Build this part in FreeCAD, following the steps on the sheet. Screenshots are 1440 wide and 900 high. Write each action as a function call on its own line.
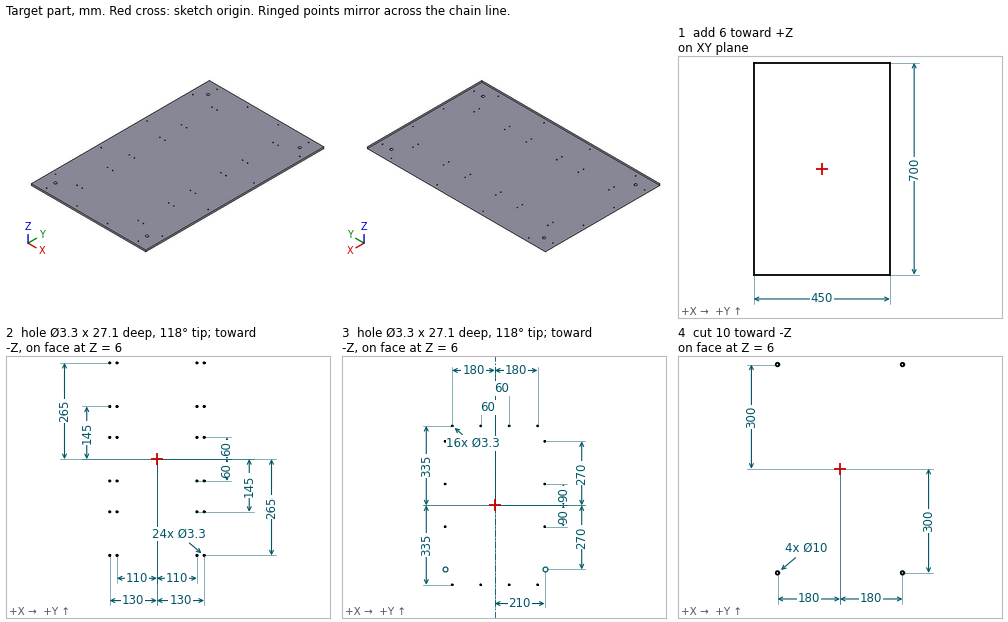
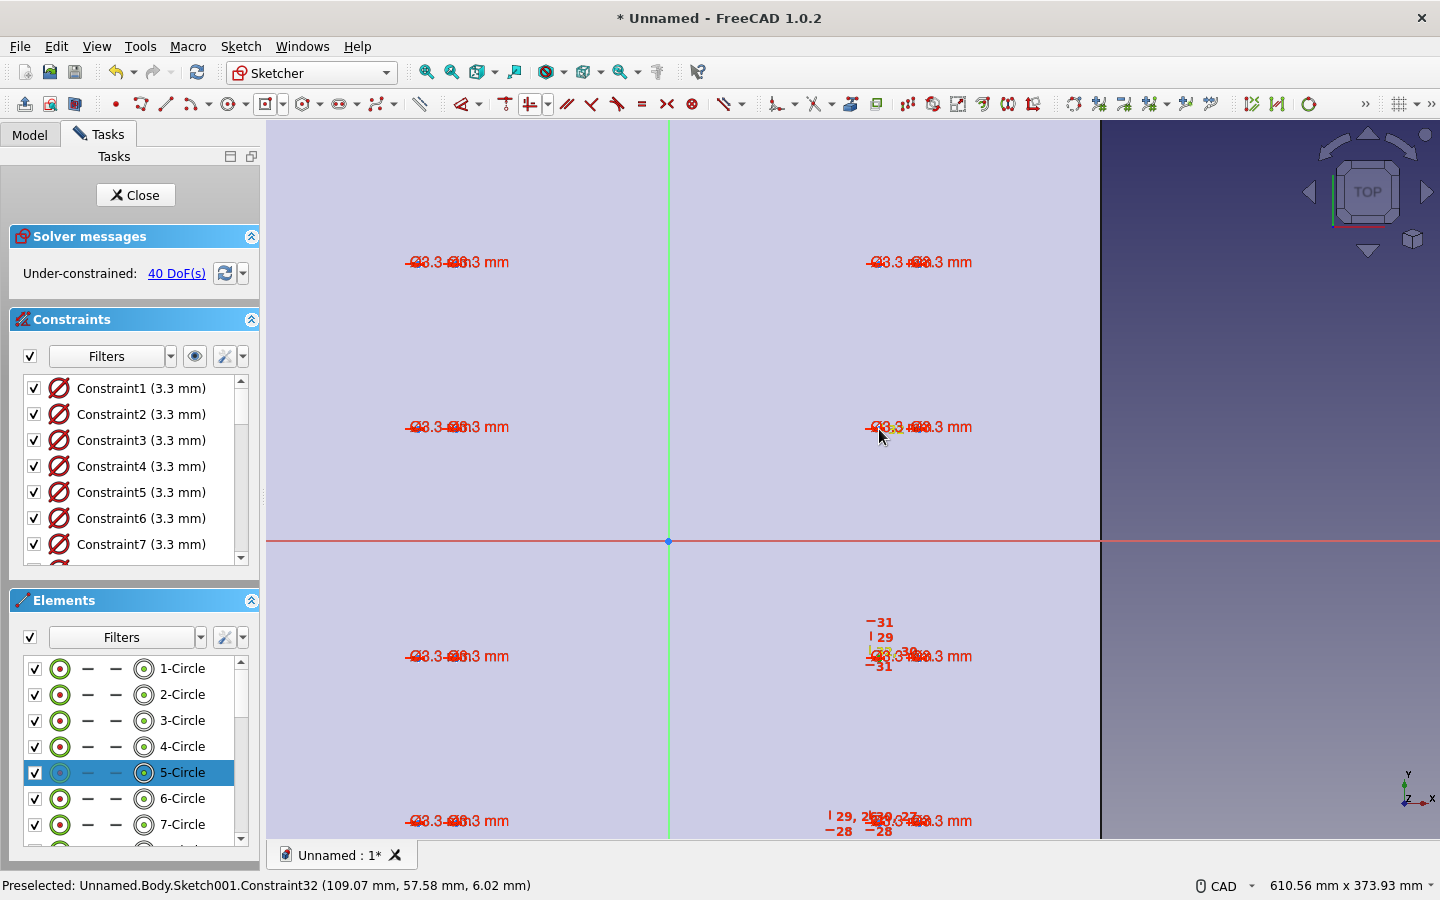
scroll(879, 429, up, 4)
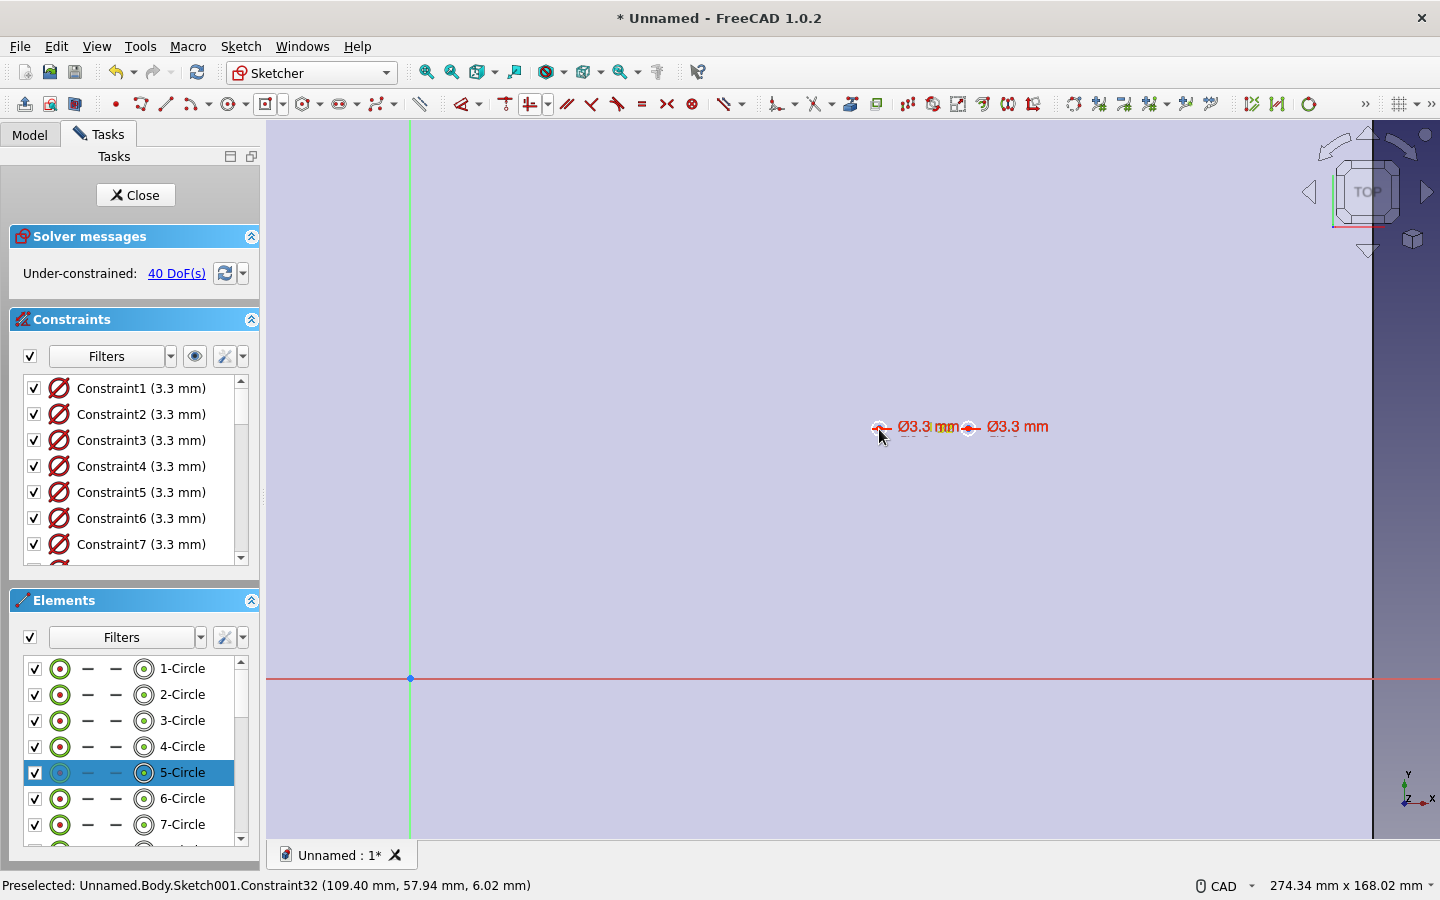
click(879, 429)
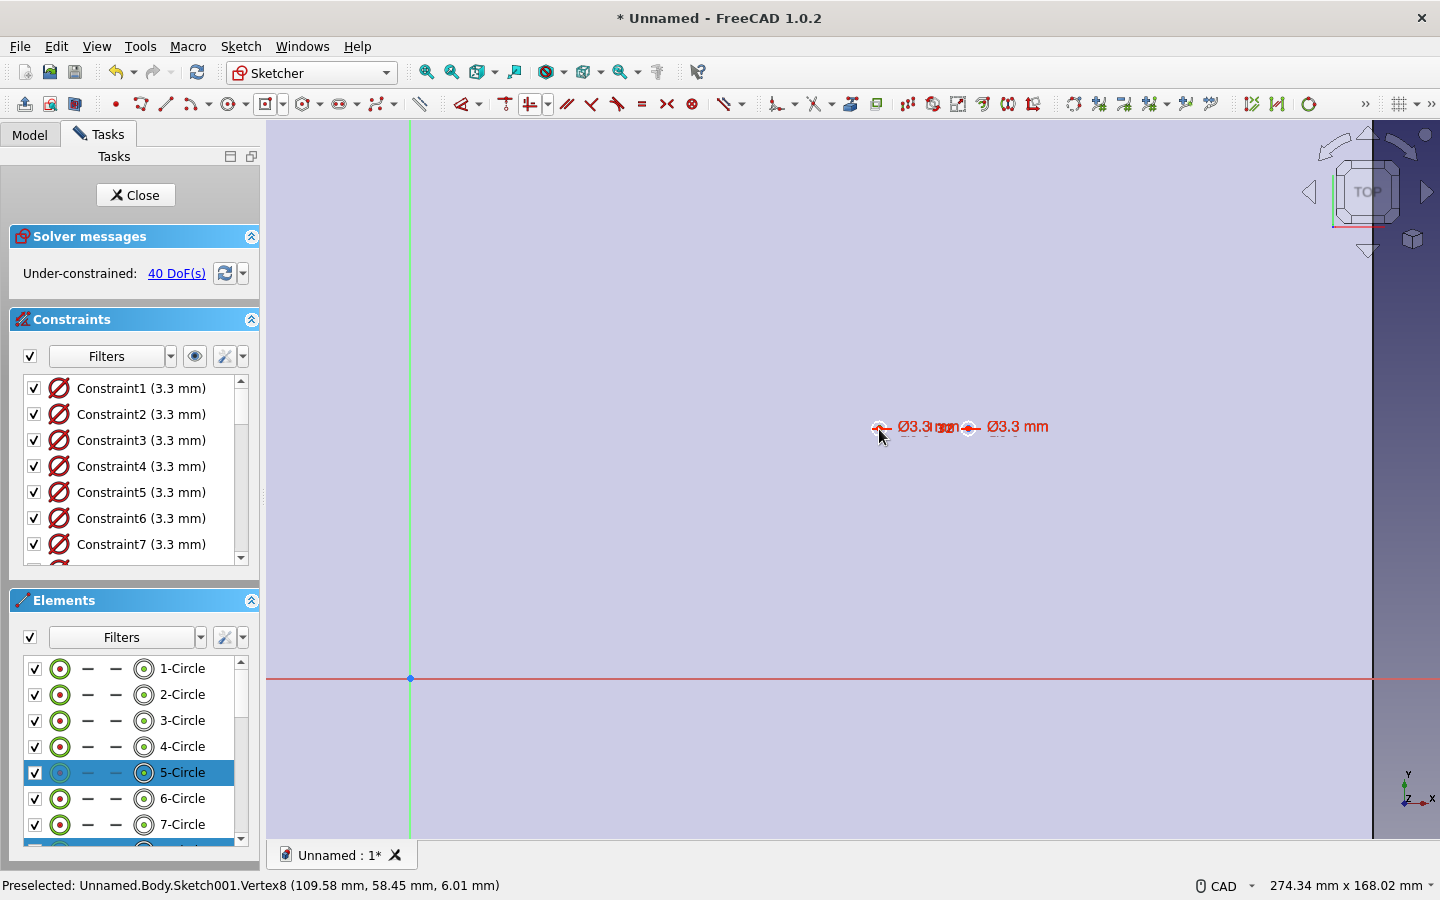
key(v)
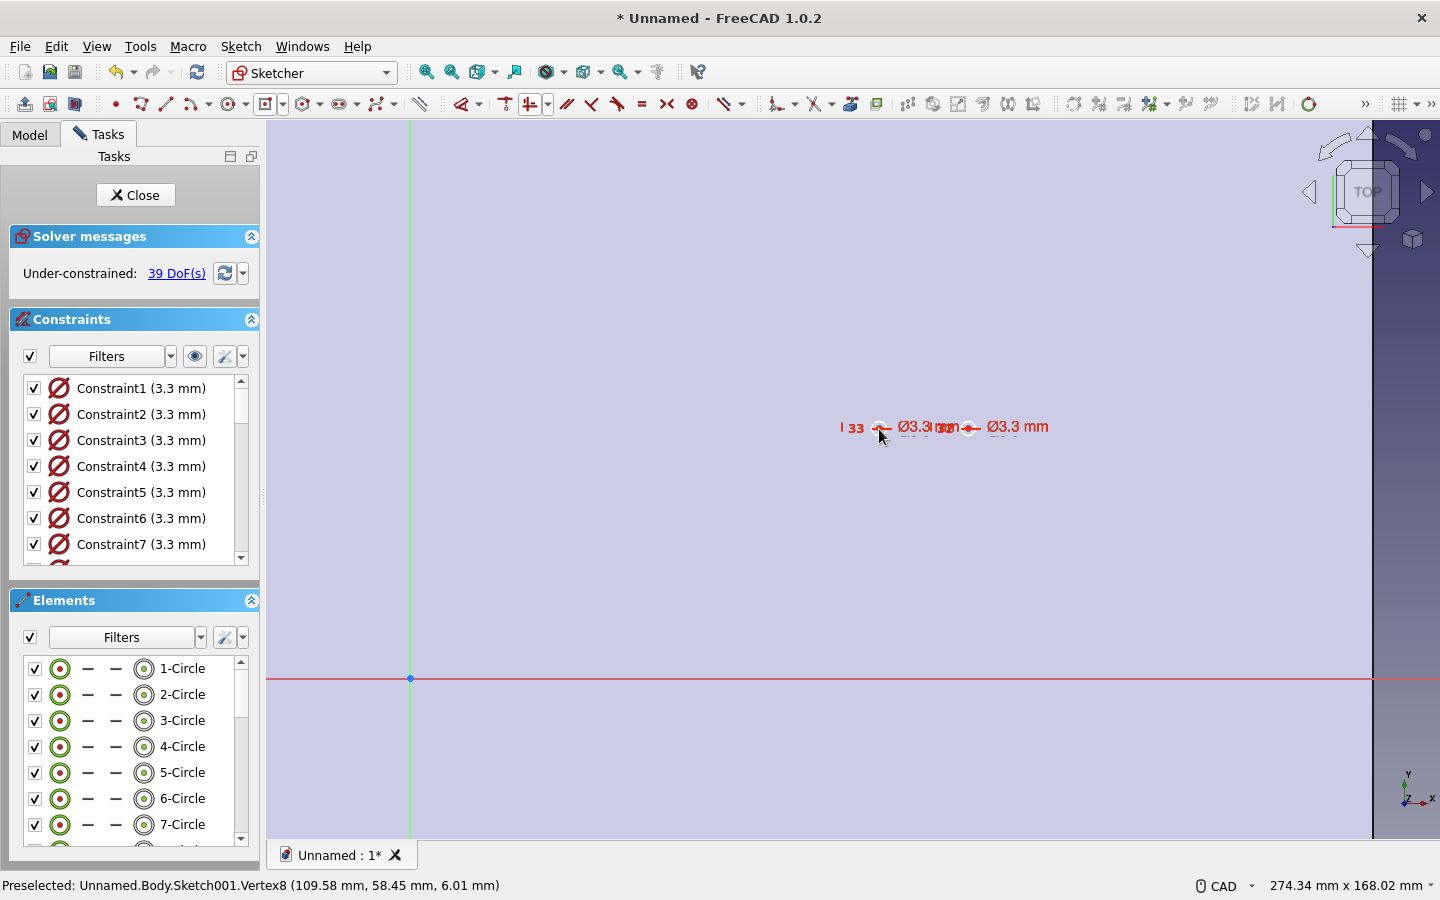
scroll(879, 429, down, 8)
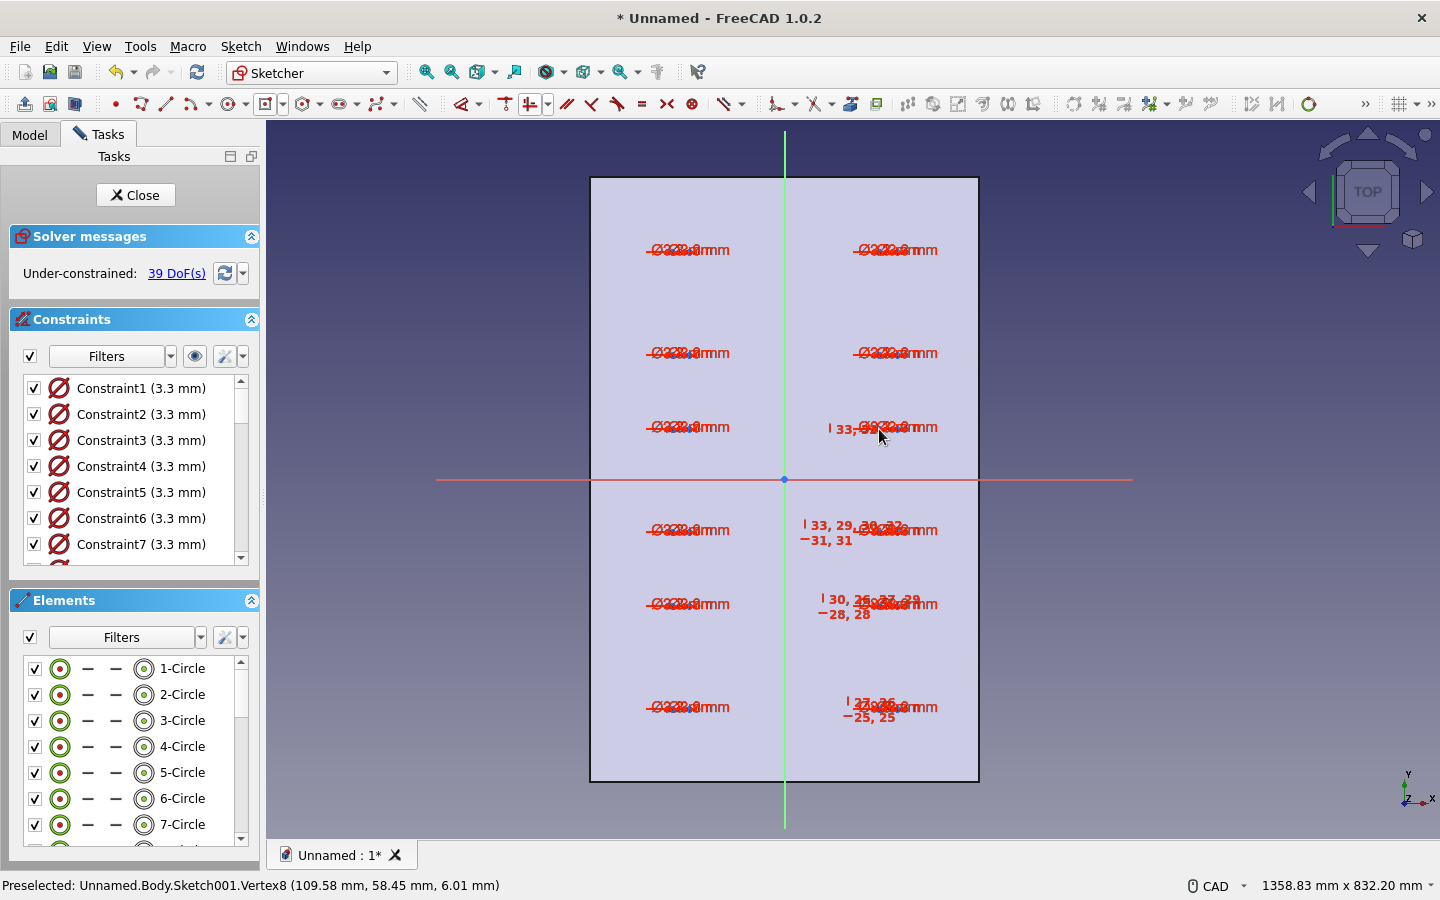
click(897, 429)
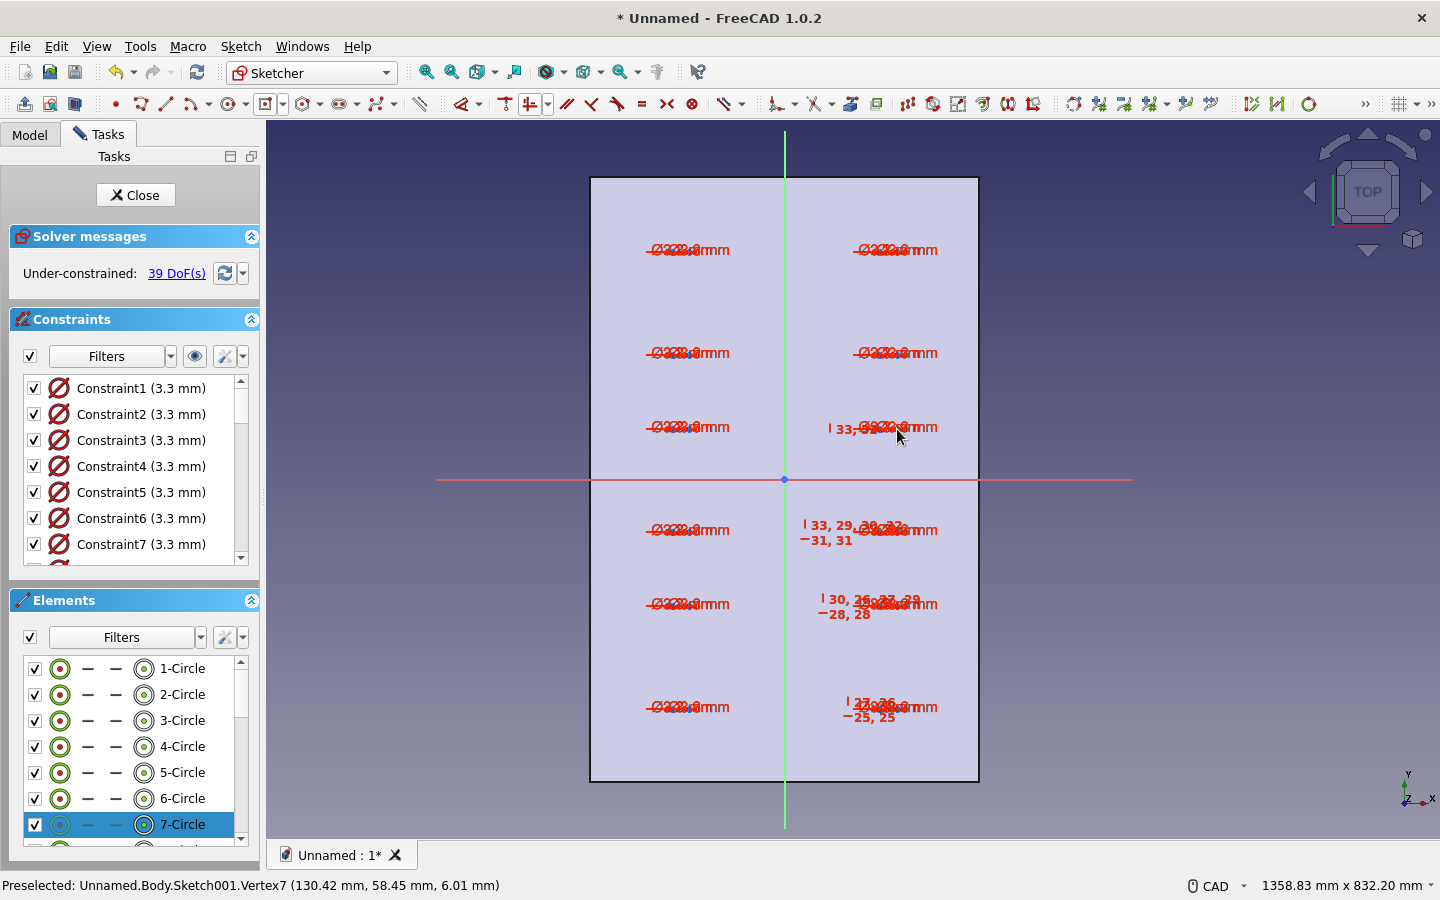
click(879, 429)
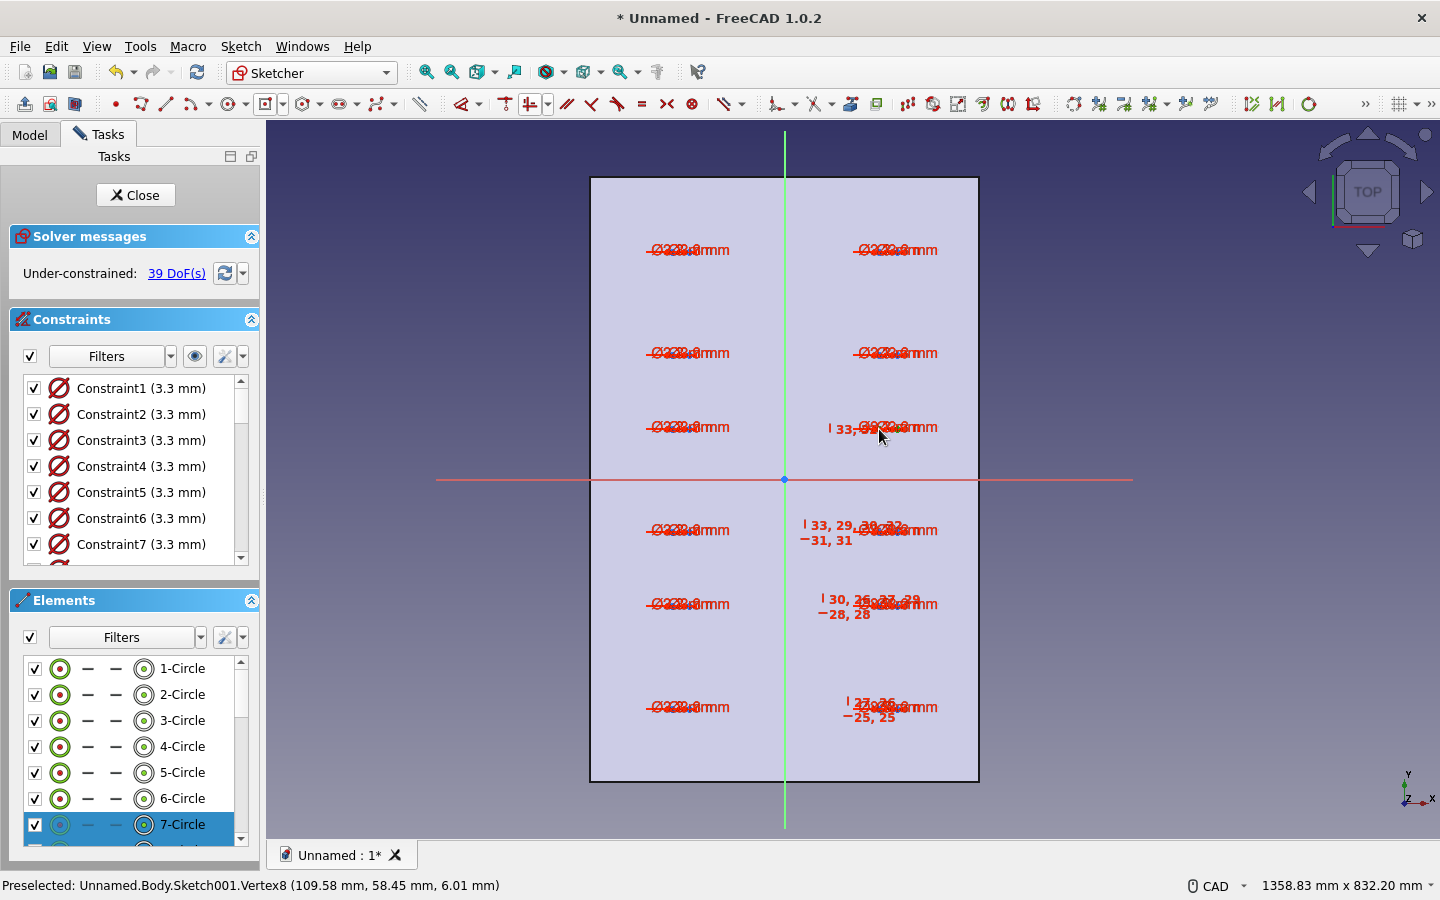
click(548, 104)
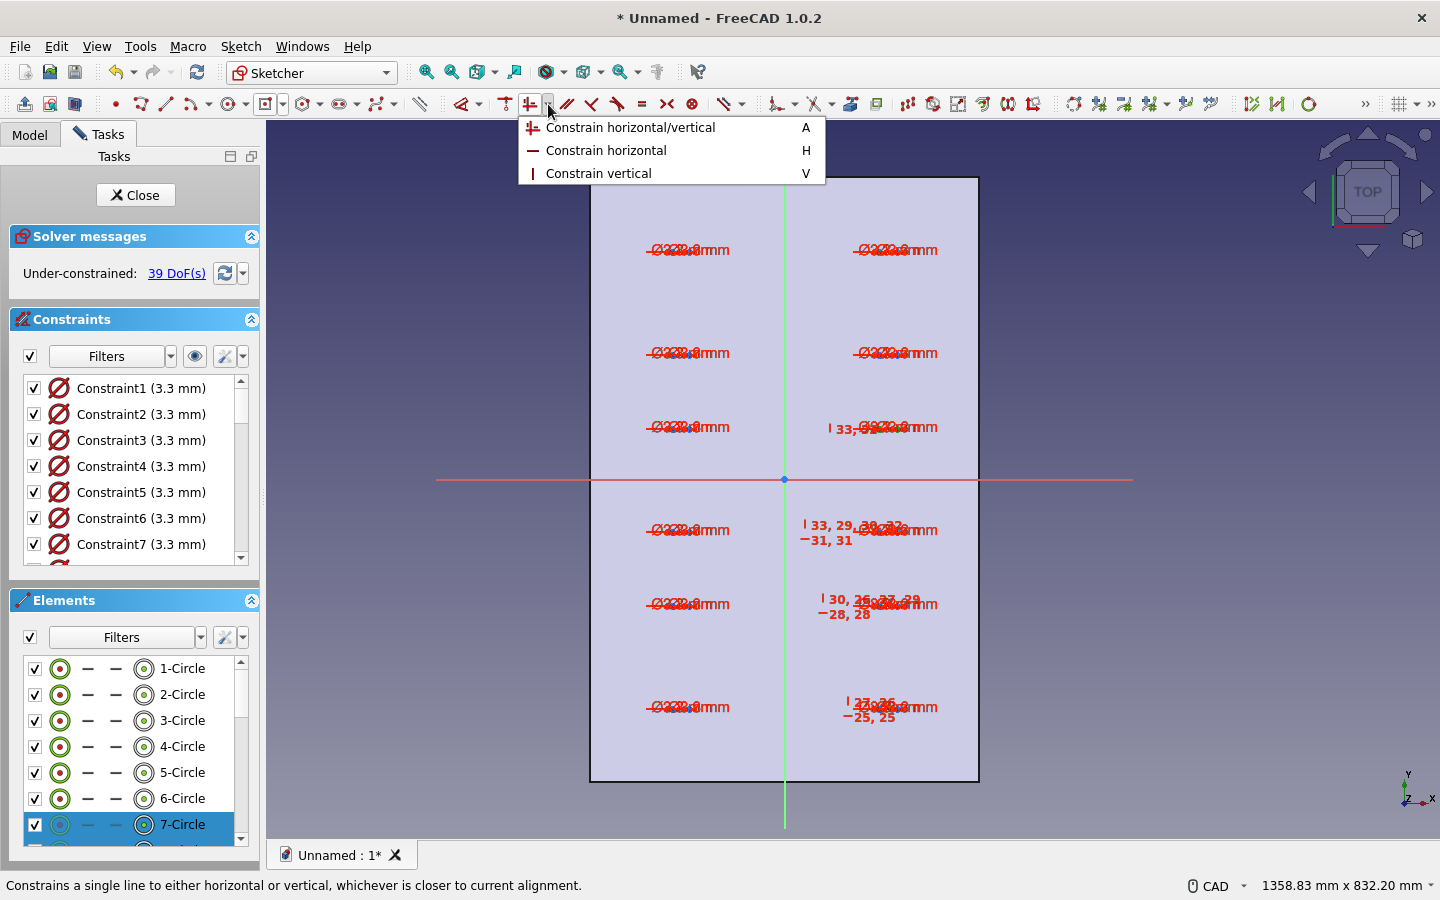
click(672, 150)